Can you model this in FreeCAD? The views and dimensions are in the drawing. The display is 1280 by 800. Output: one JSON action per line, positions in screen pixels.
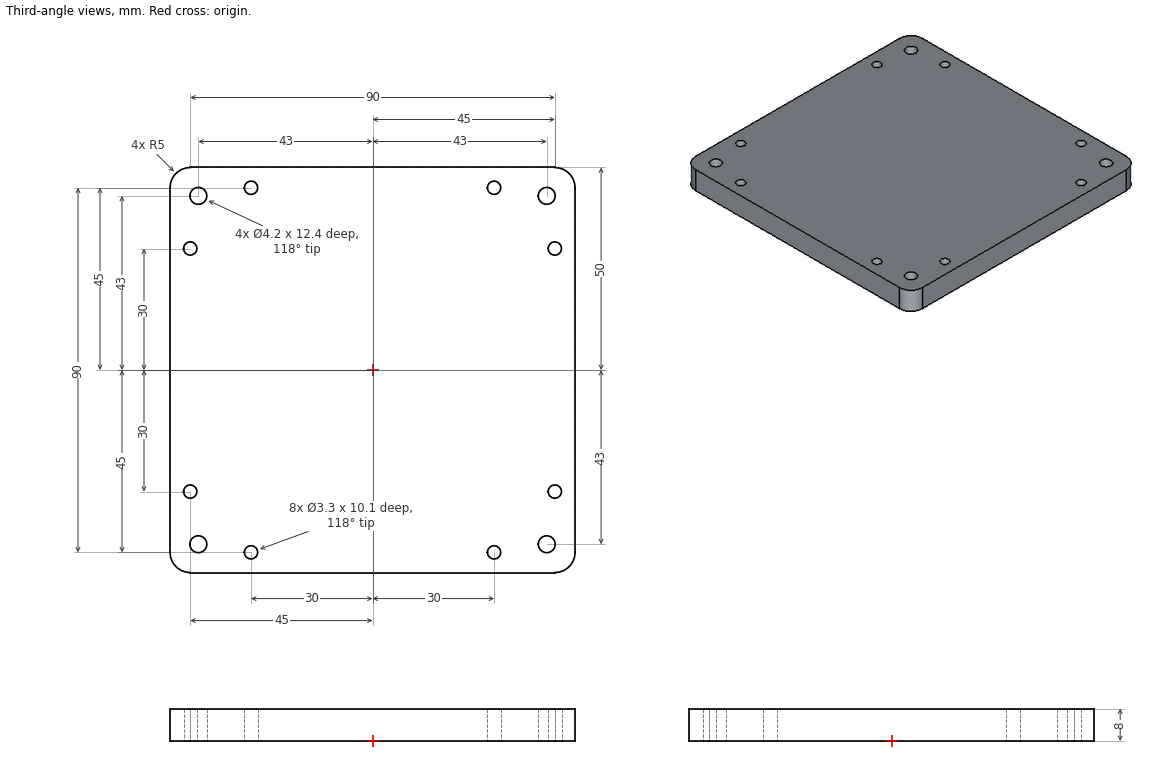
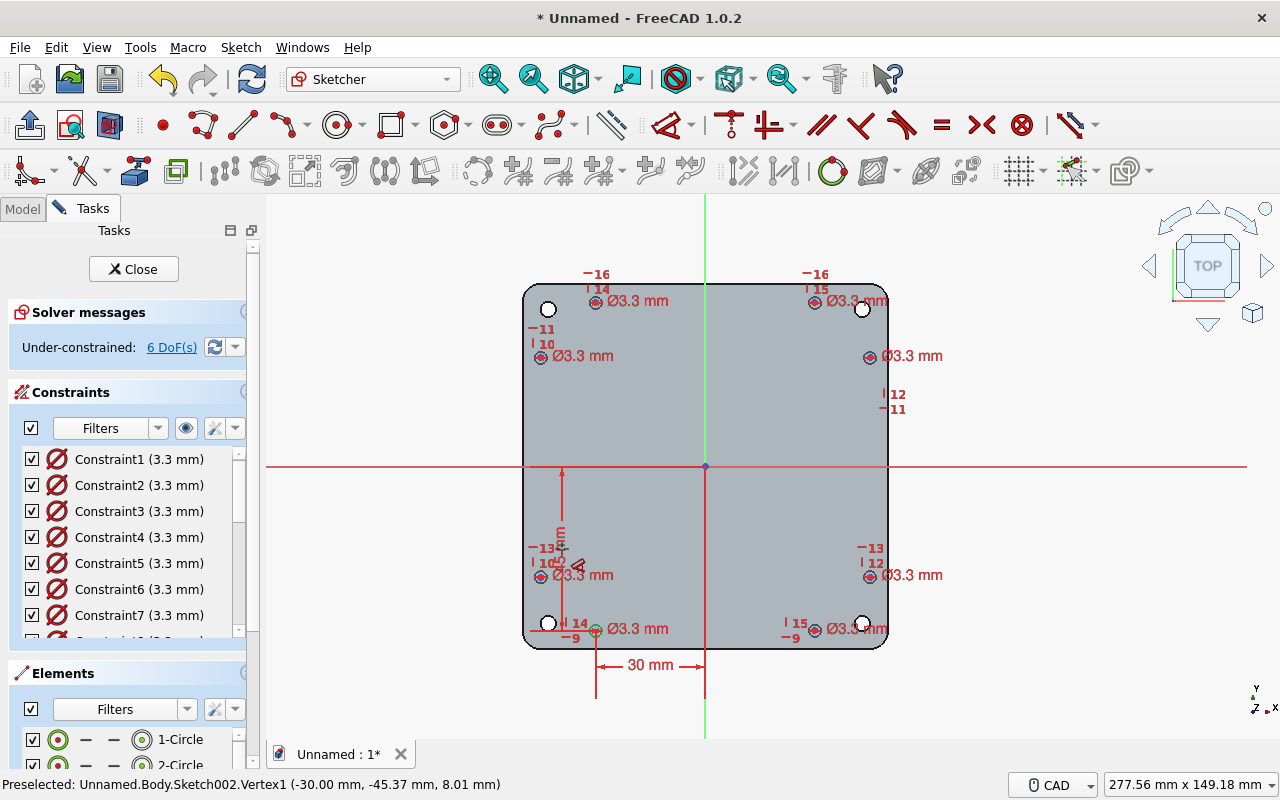
{"action": "left_click", "coordinate": [815, 631]}
{"action": "left_click", "coordinate": [760, 665]}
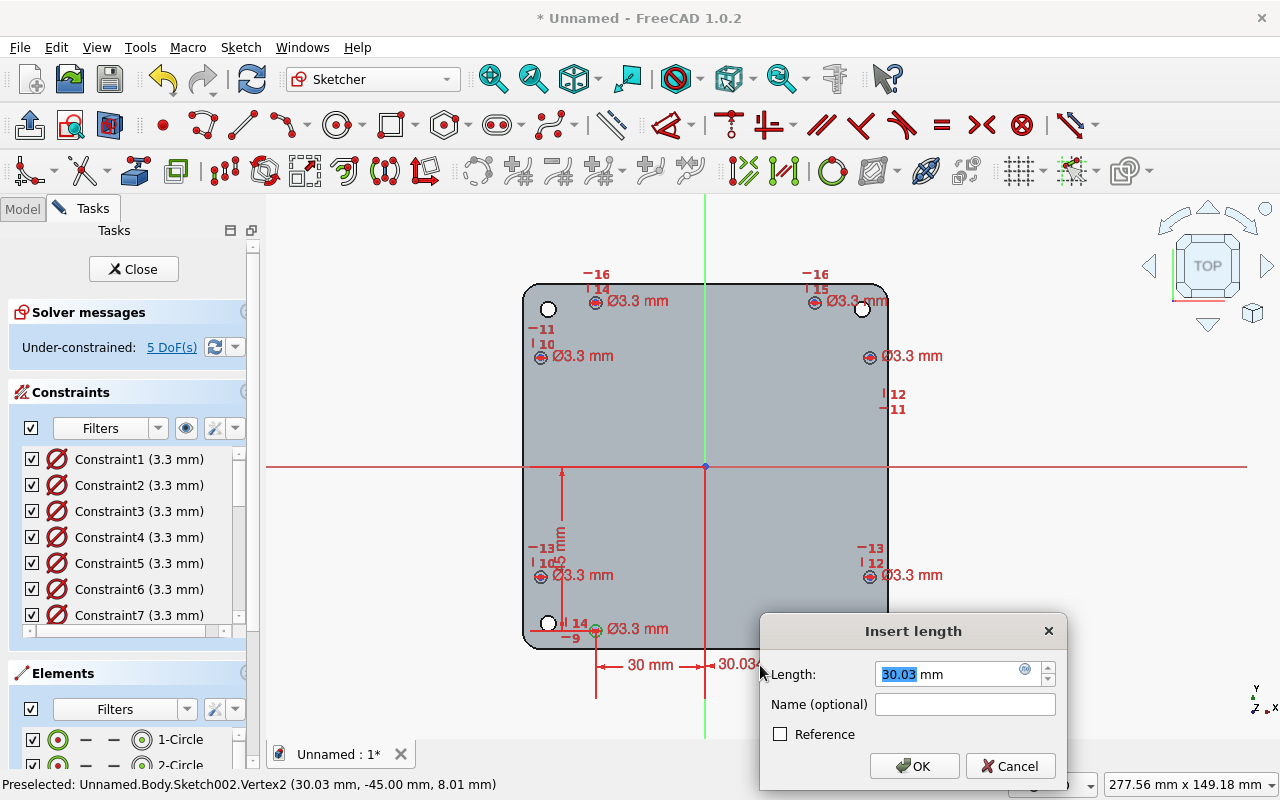
{"action": "type", "text": "30"}
{"action": "key", "text": "Return"}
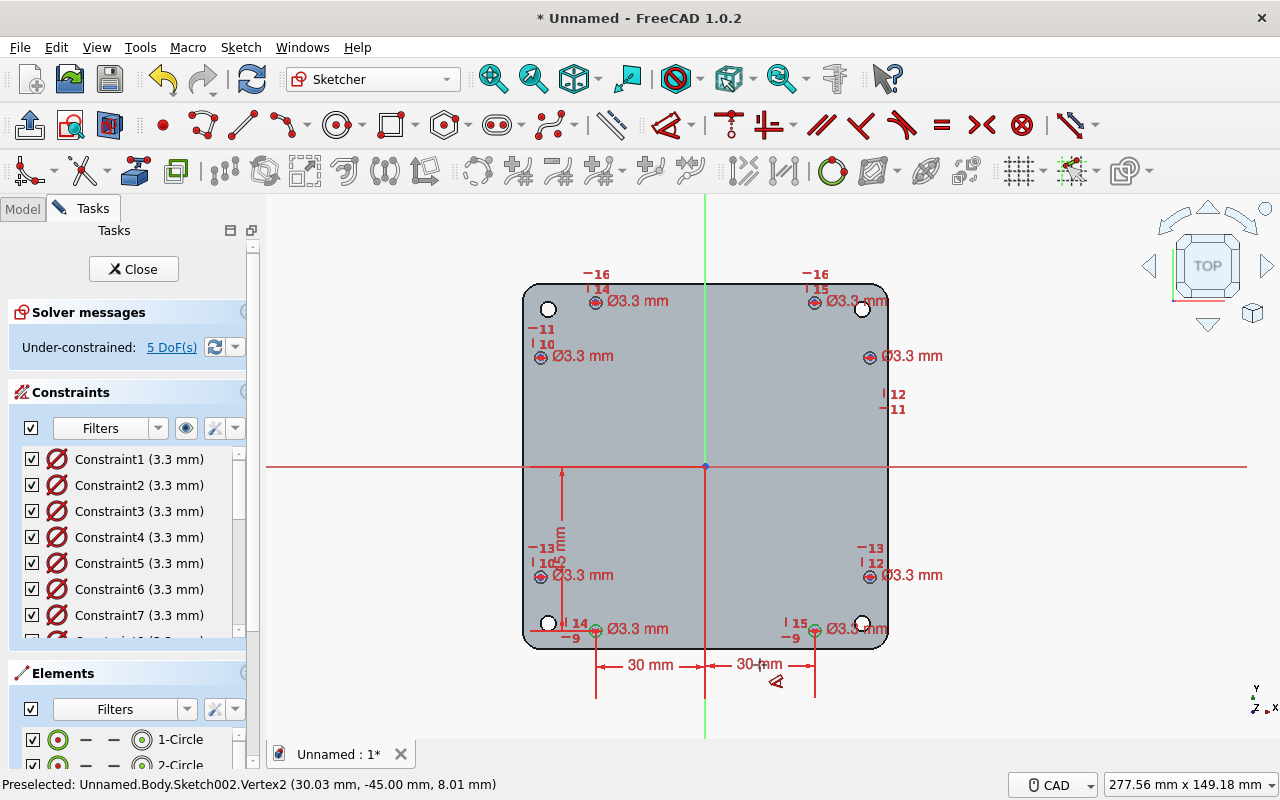
{"action": "left_click", "coordinate": [541, 577]}
{"action": "left_click", "coordinate": [623, 611]}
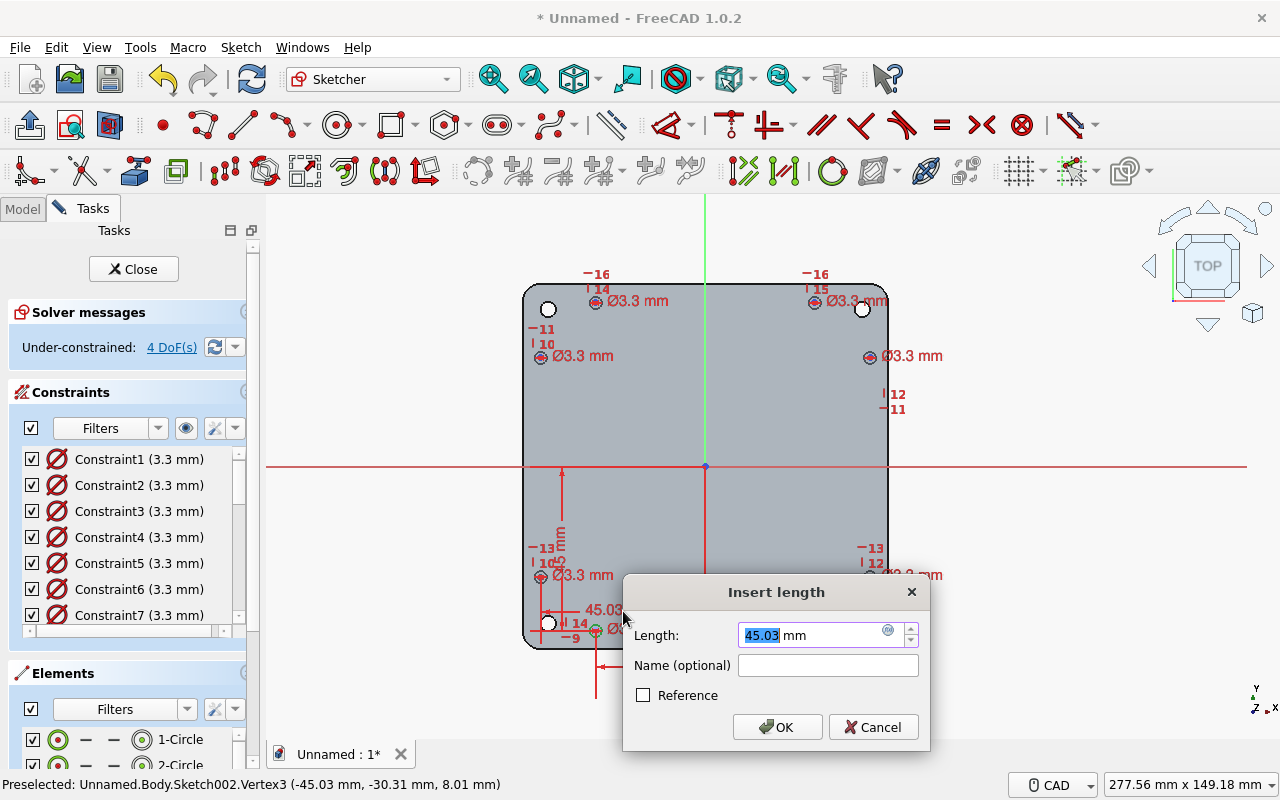
{"action": "type", "text": "45"}
{"action": "key", "text": "Return"}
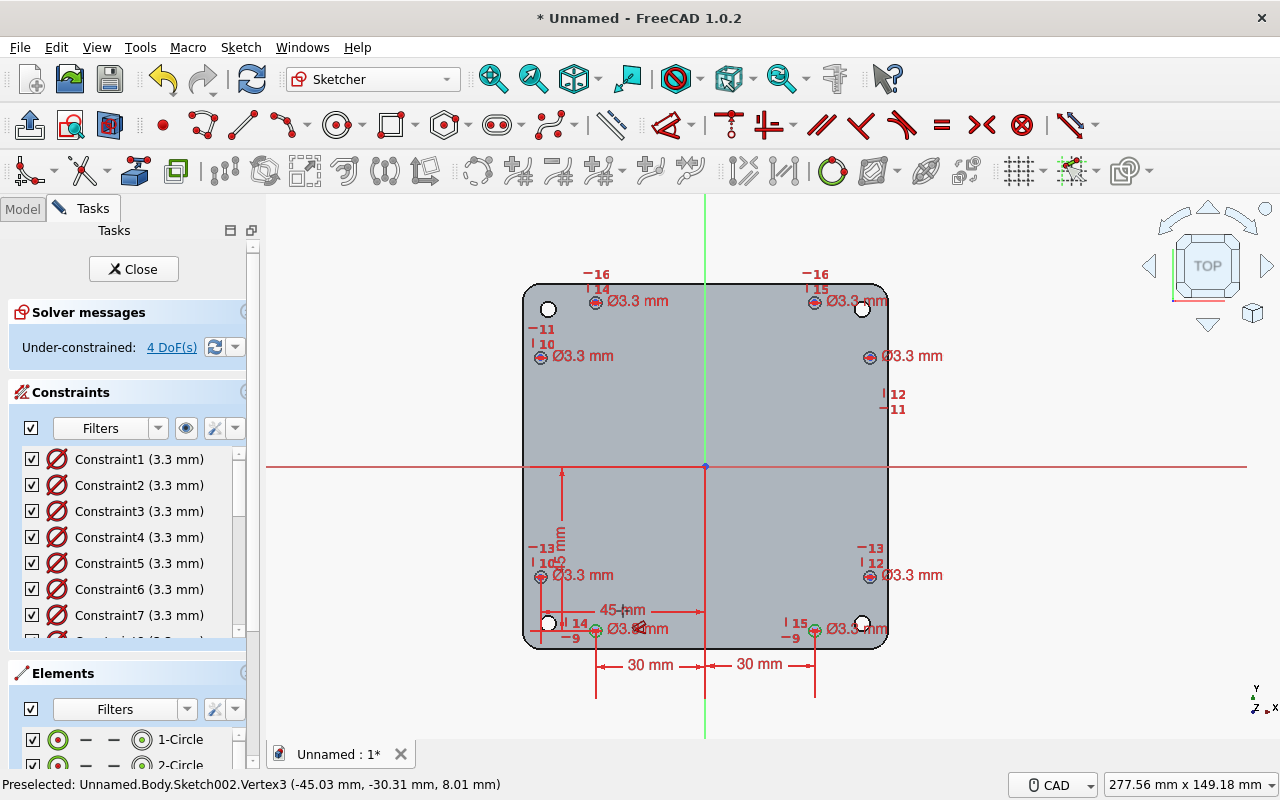
{"action": "left_click", "coordinate": [541, 577]}
{"action": "left_click", "coordinate": [507, 522]}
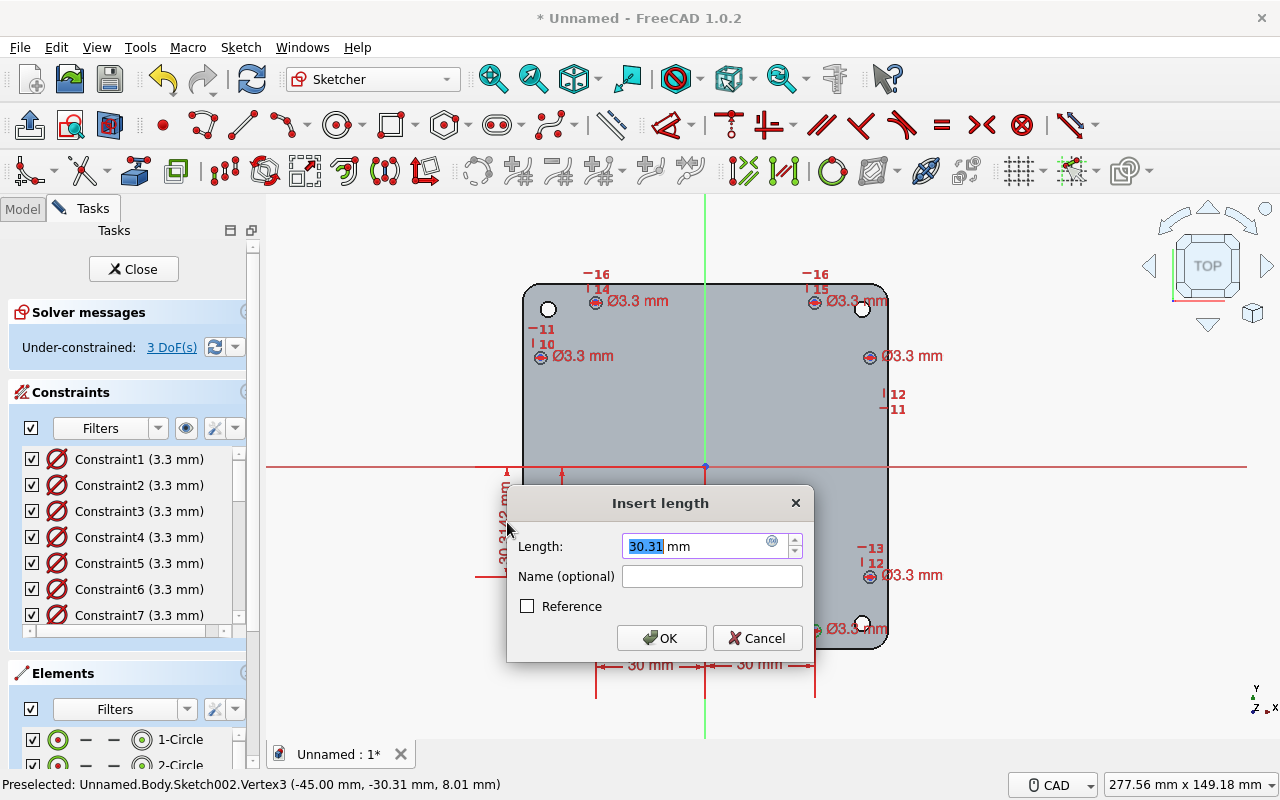
{"action": "type", "text": "30"}
{"action": "key", "text": "Return"}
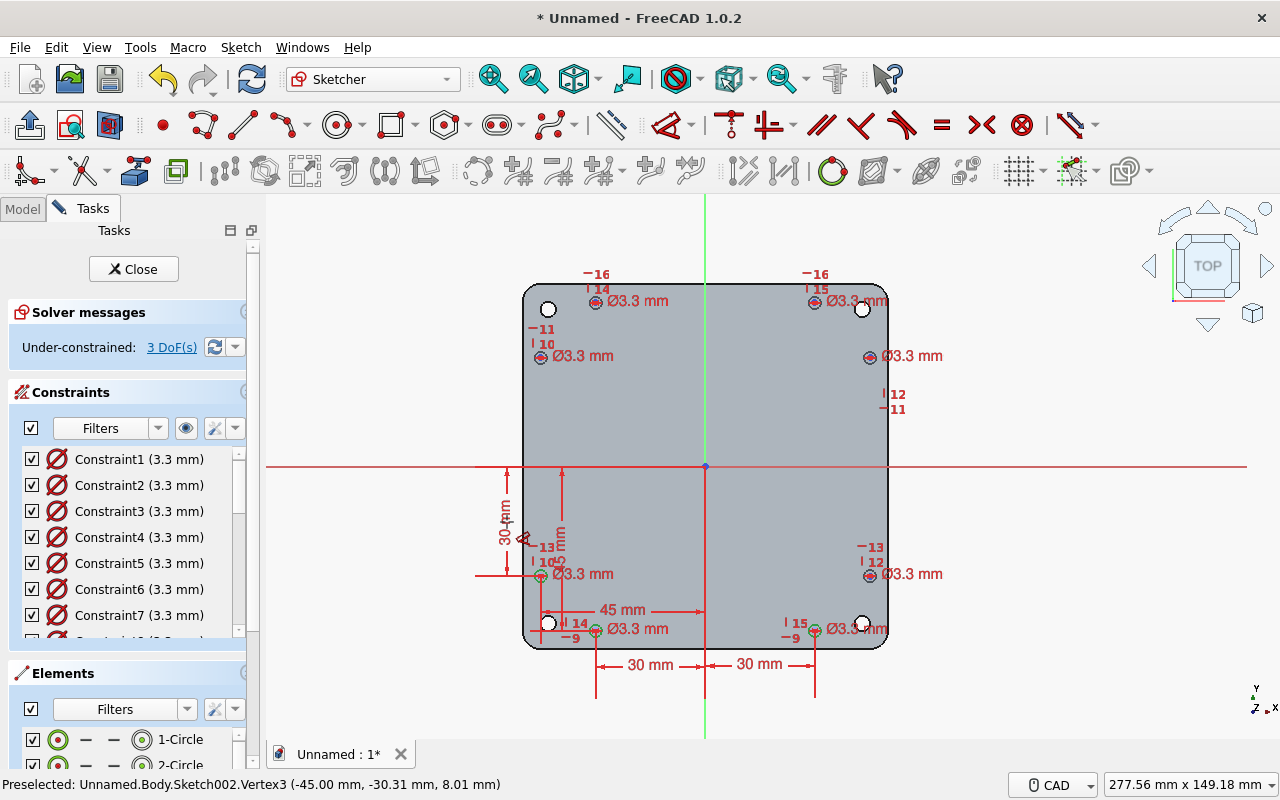
{"action": "left_click", "coordinate": [541, 358]}
{"action": "left_click", "coordinate": [507, 412]}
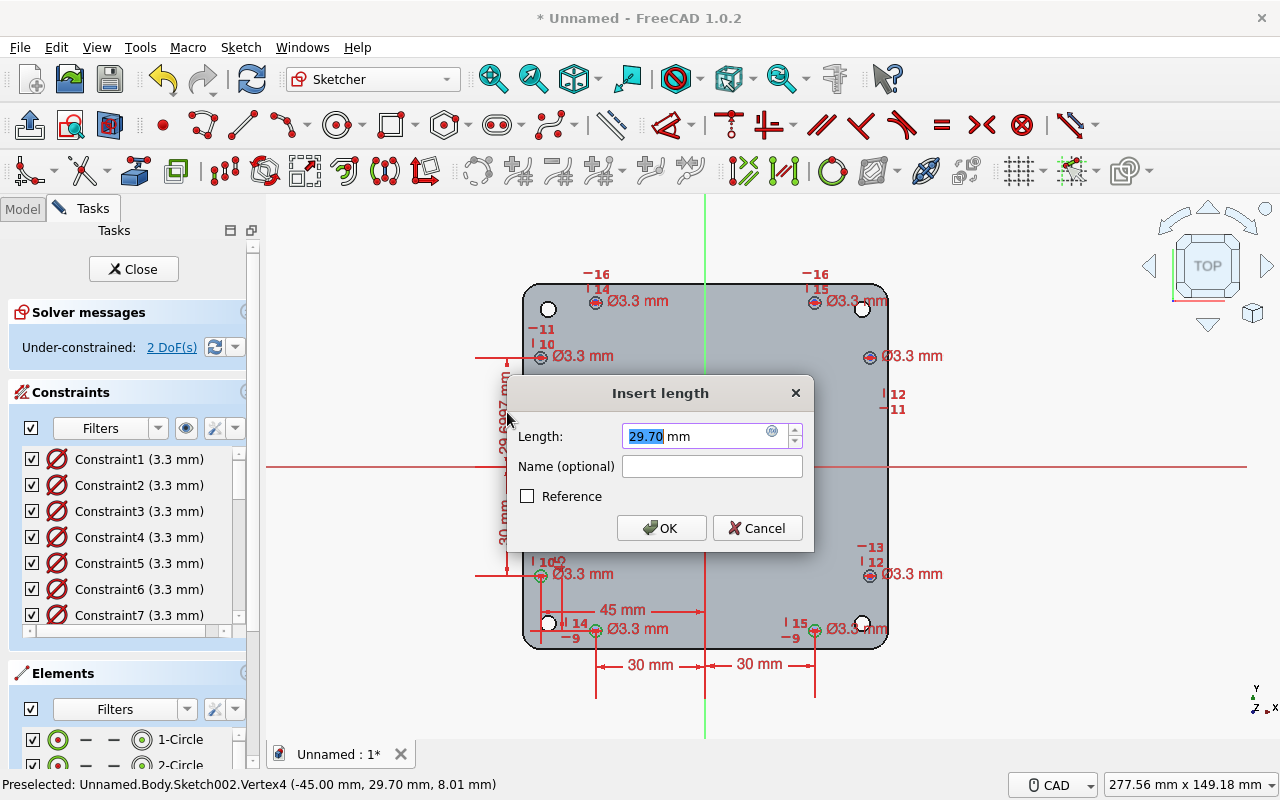
{"action": "type", "text": "30"}
{"action": "key", "text": "Return"}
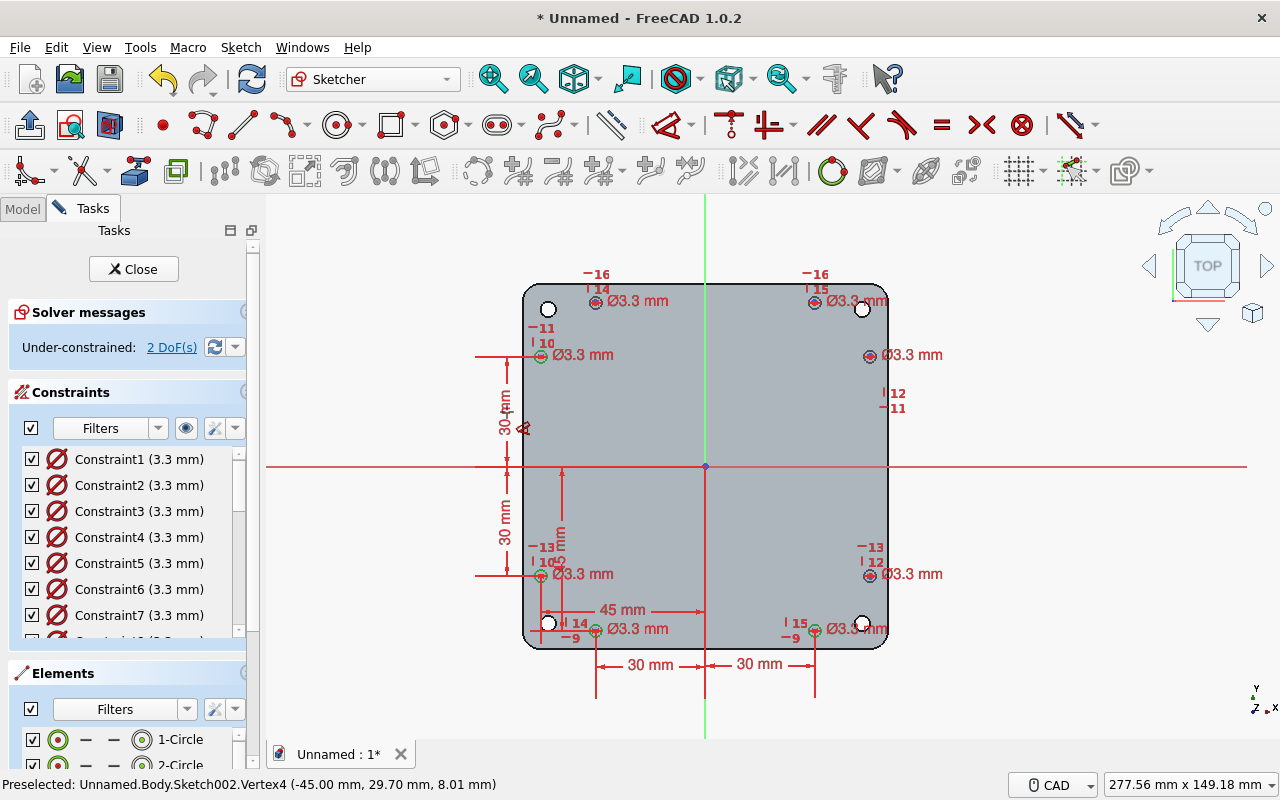
{"action": "left_click", "coordinate": [870, 357]}
{"action": "left_click", "coordinate": [788, 323]}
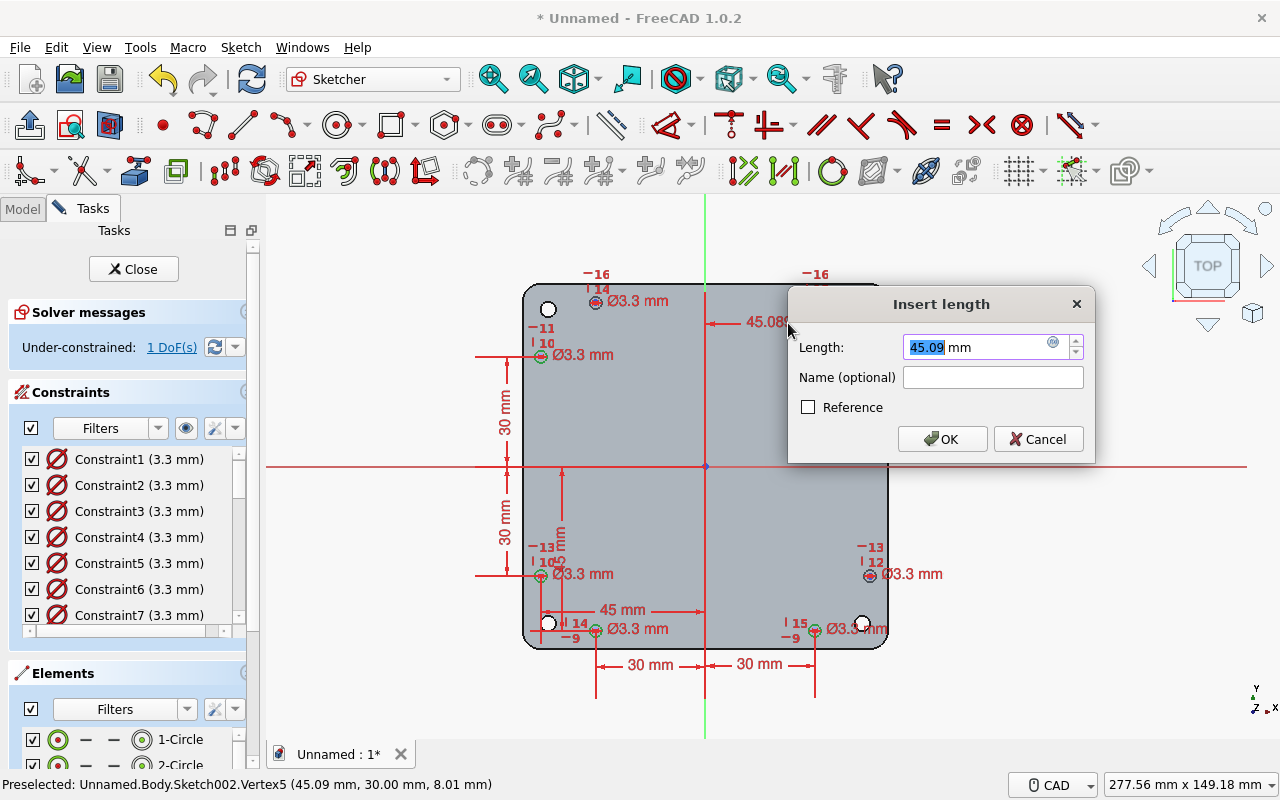
{"action": "type", "text": "45"}
{"action": "key", "text": "Return"}